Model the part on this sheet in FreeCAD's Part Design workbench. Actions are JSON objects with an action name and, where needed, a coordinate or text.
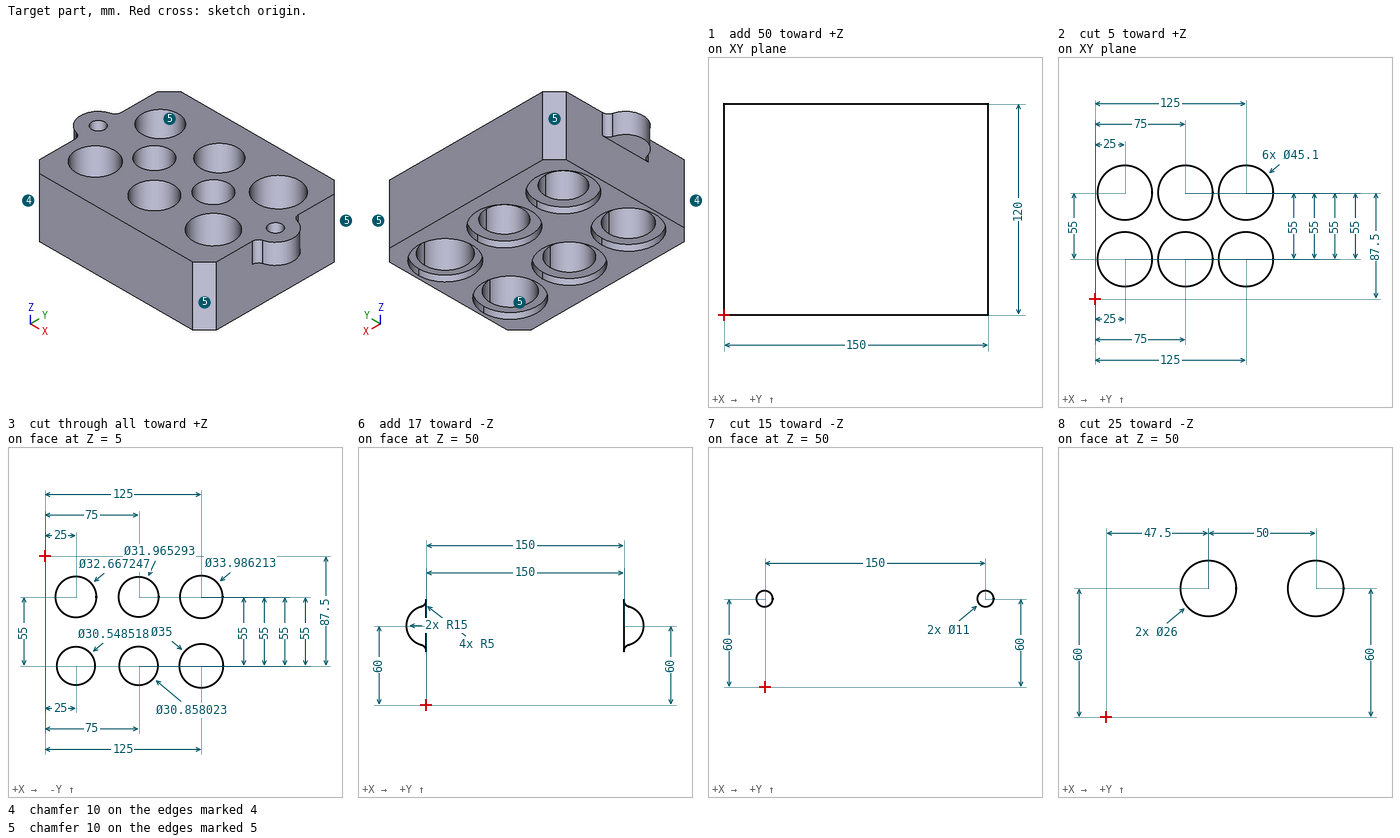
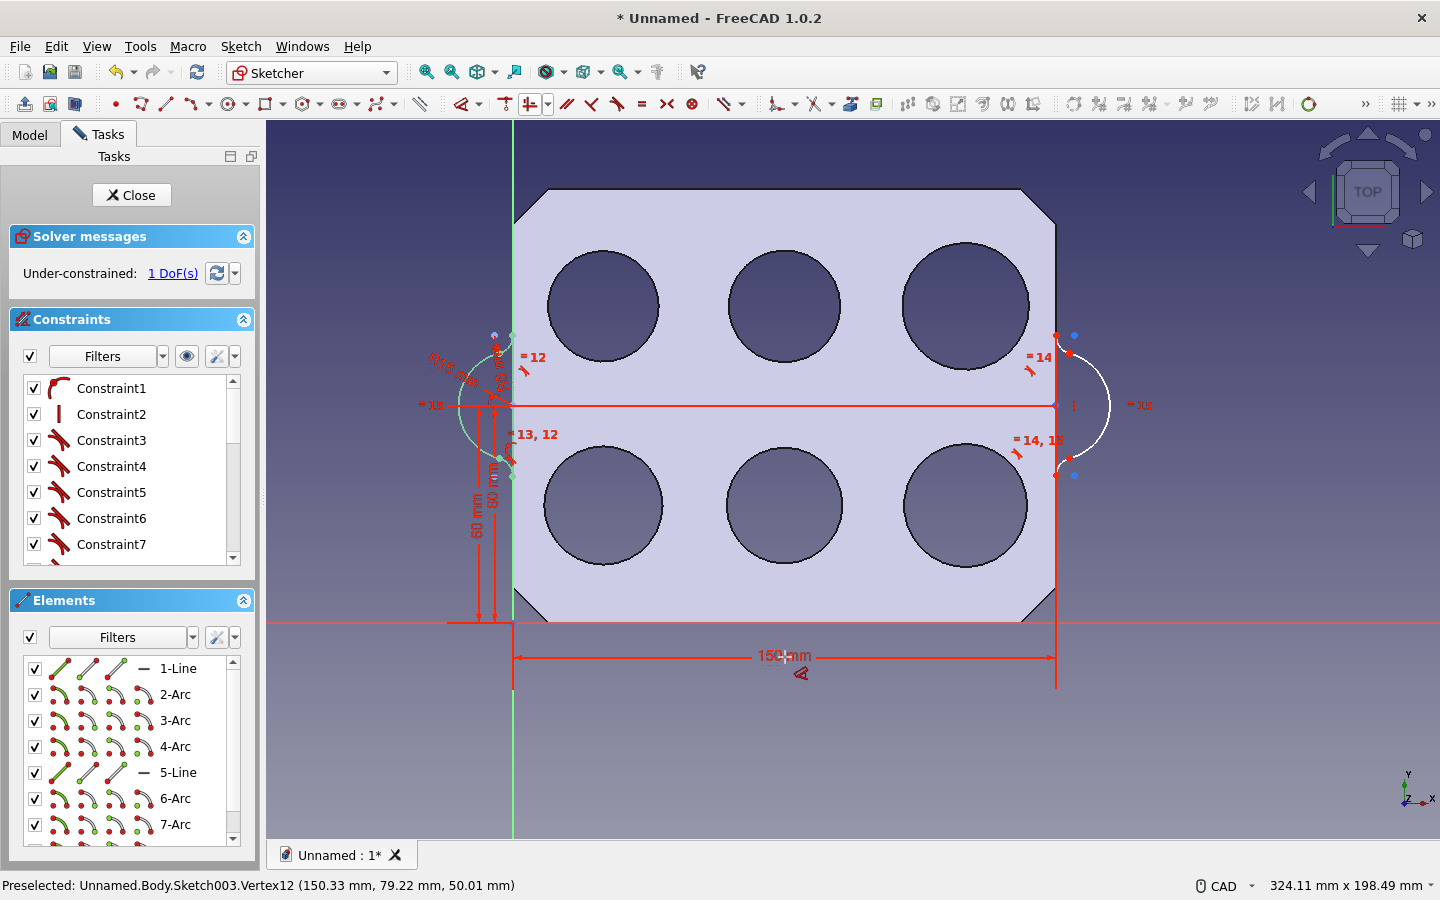
{"action": "left_click", "coordinate": [1055, 406]}
{"action": "left_click", "coordinate": [659, 657]}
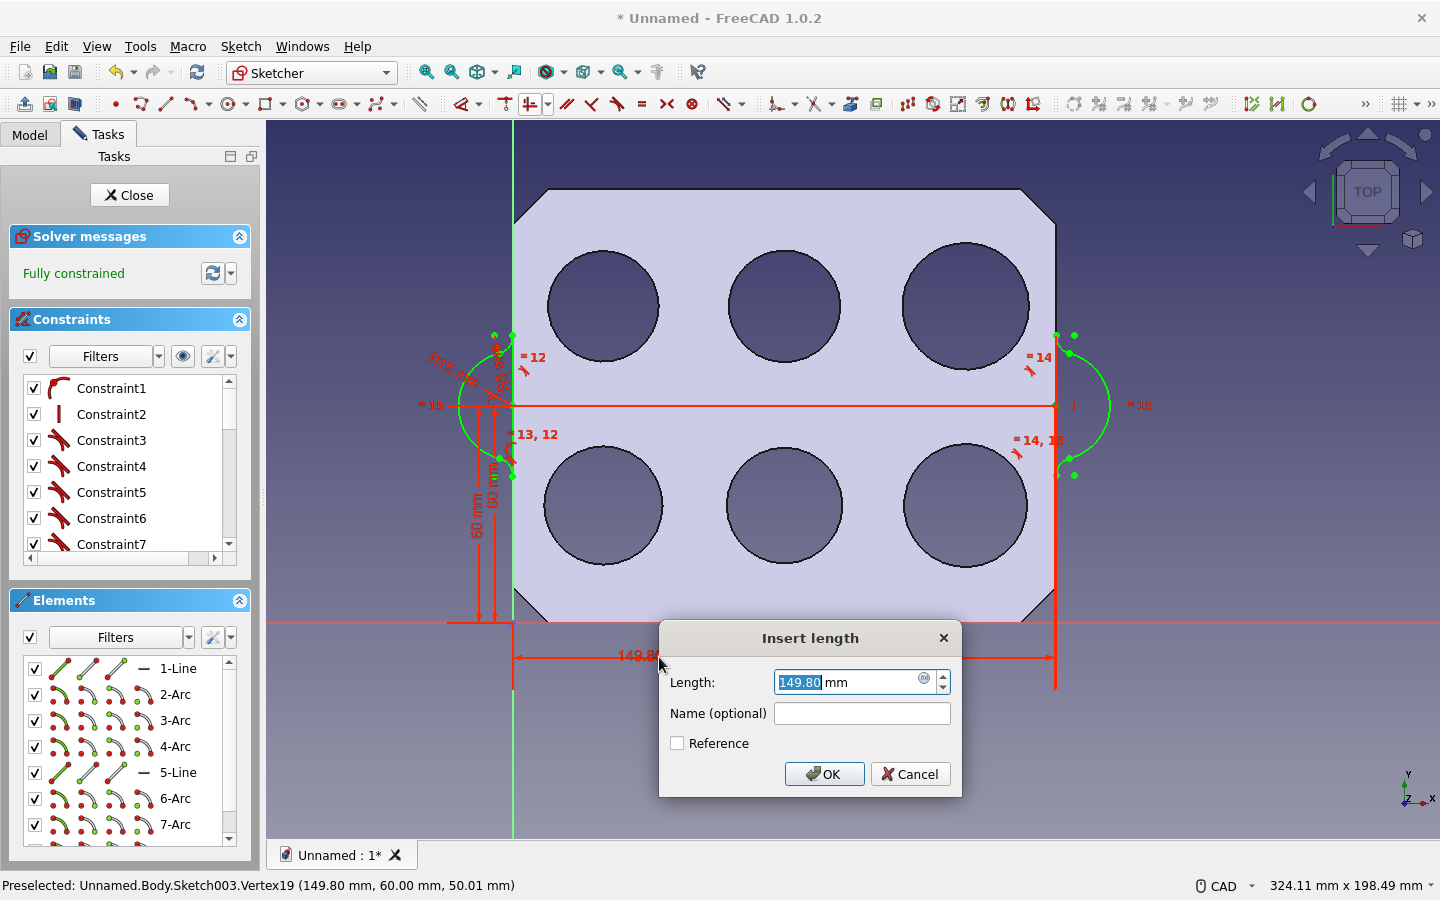
{"action": "type", "text": "150"}
{"action": "key", "text": "Return"}
{"action": "key", "text": "Escape"}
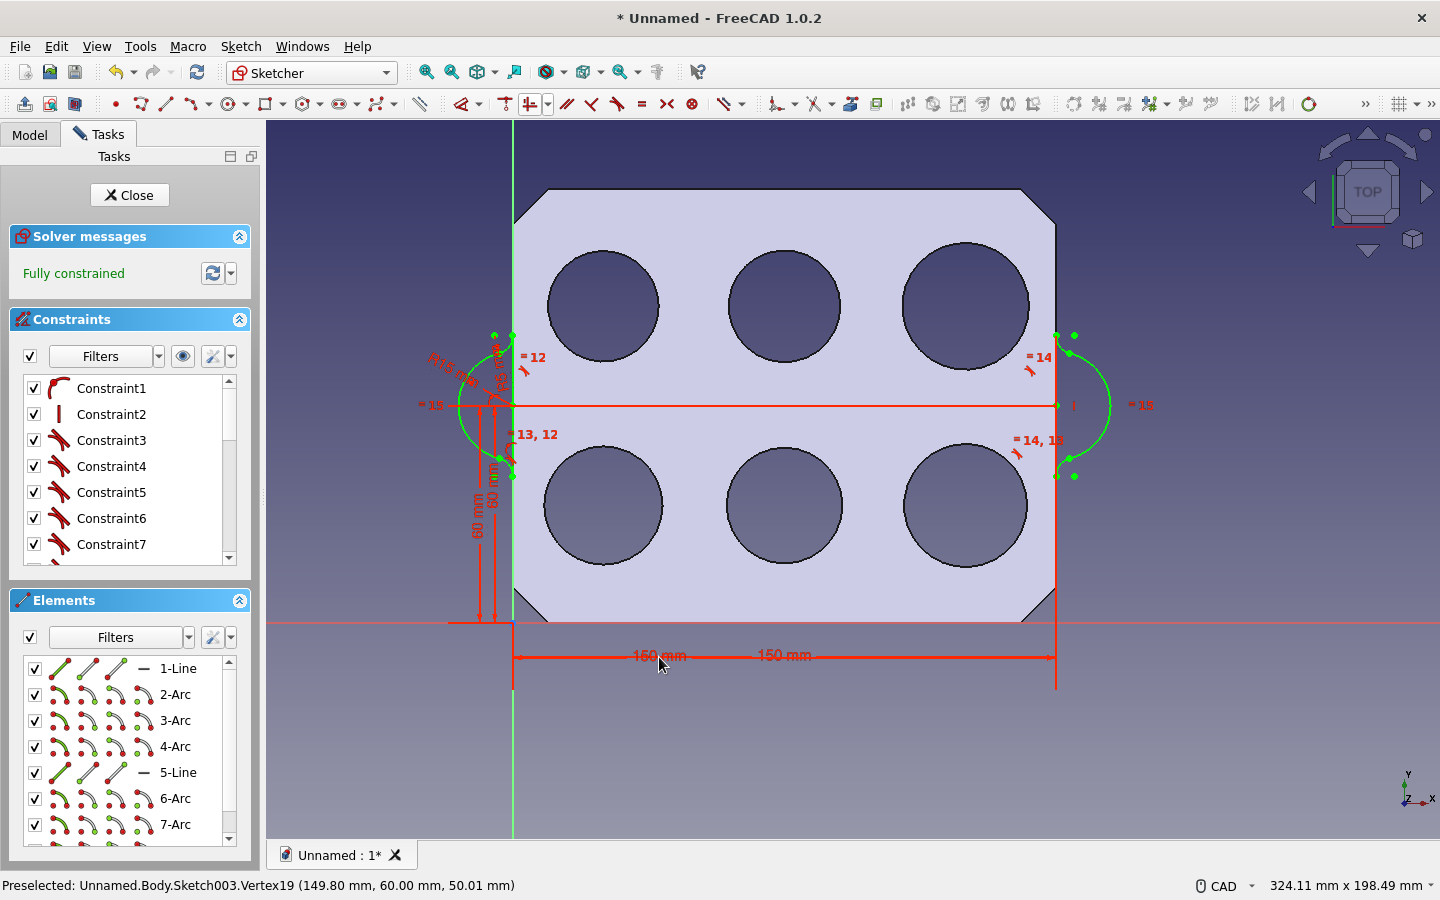
{"action": "left_click", "coordinate": [130, 195]}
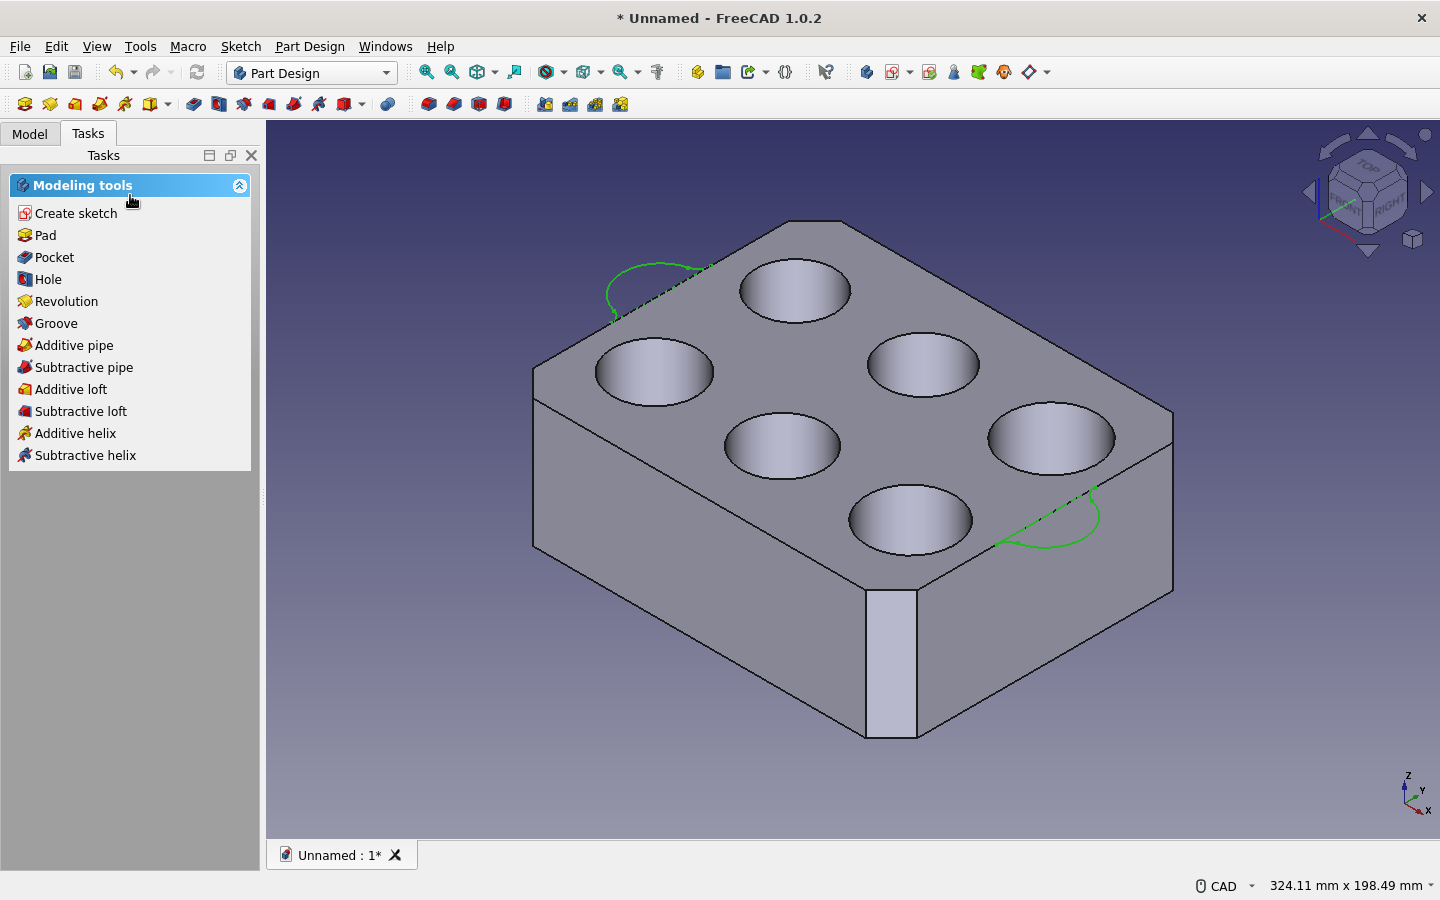
{"action": "left_click", "coordinate": [25, 104]}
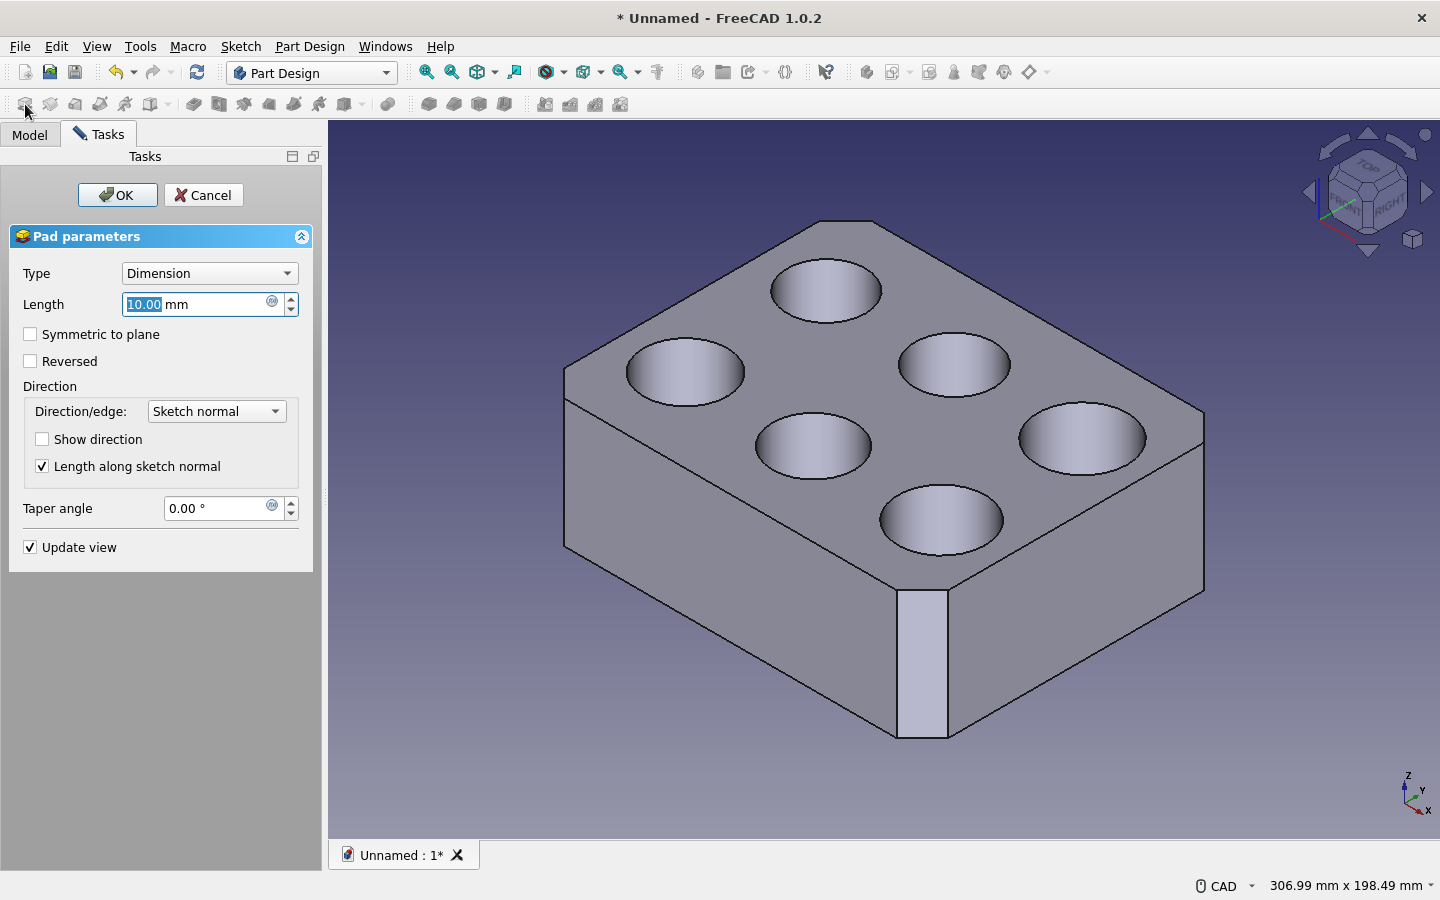
{"action": "type", "text": "17"}
{"action": "key", "text": "Tab"}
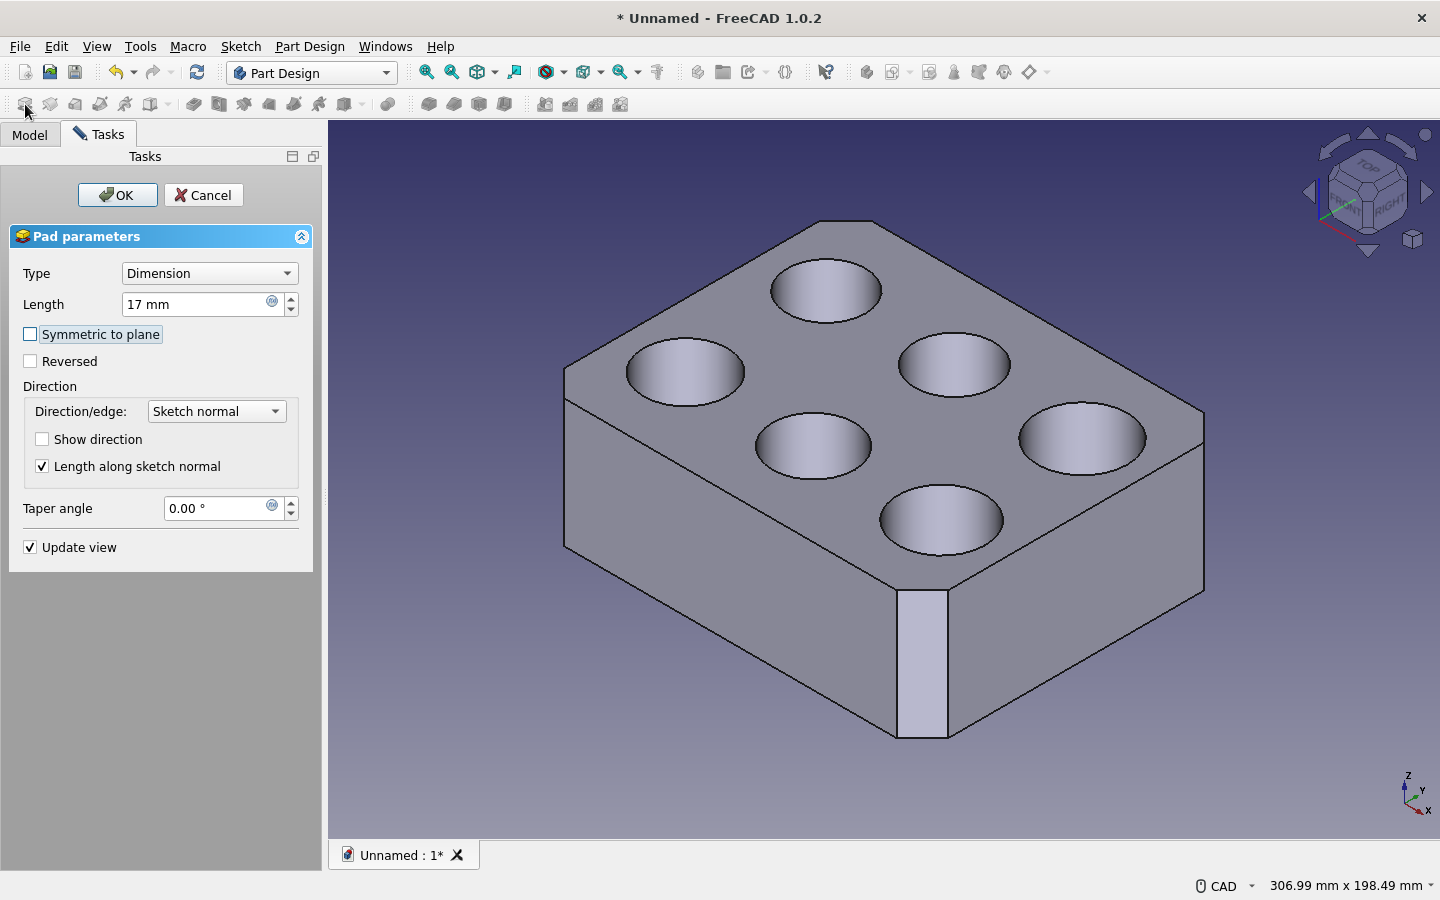
{"action": "left_click", "coordinate": [31, 361]}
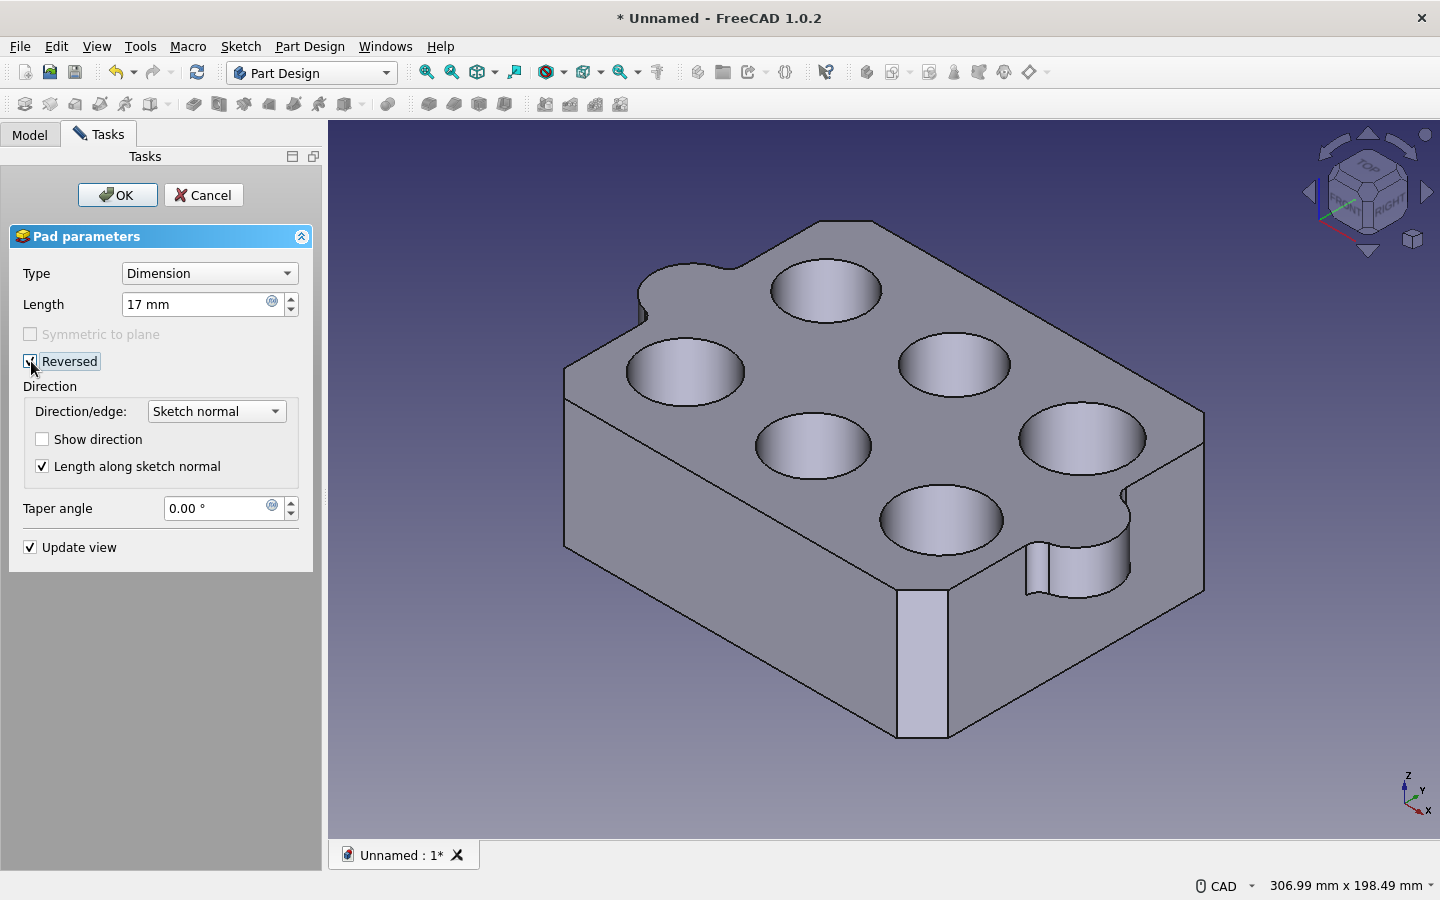
{"action": "left_click", "coordinate": [118, 195]}